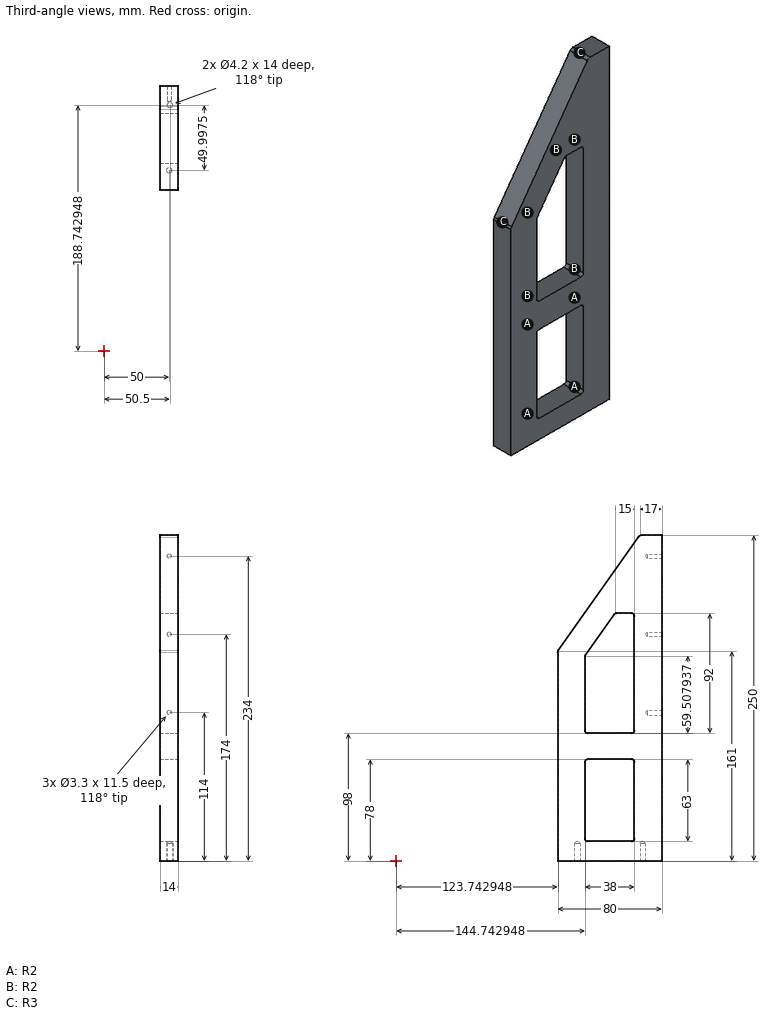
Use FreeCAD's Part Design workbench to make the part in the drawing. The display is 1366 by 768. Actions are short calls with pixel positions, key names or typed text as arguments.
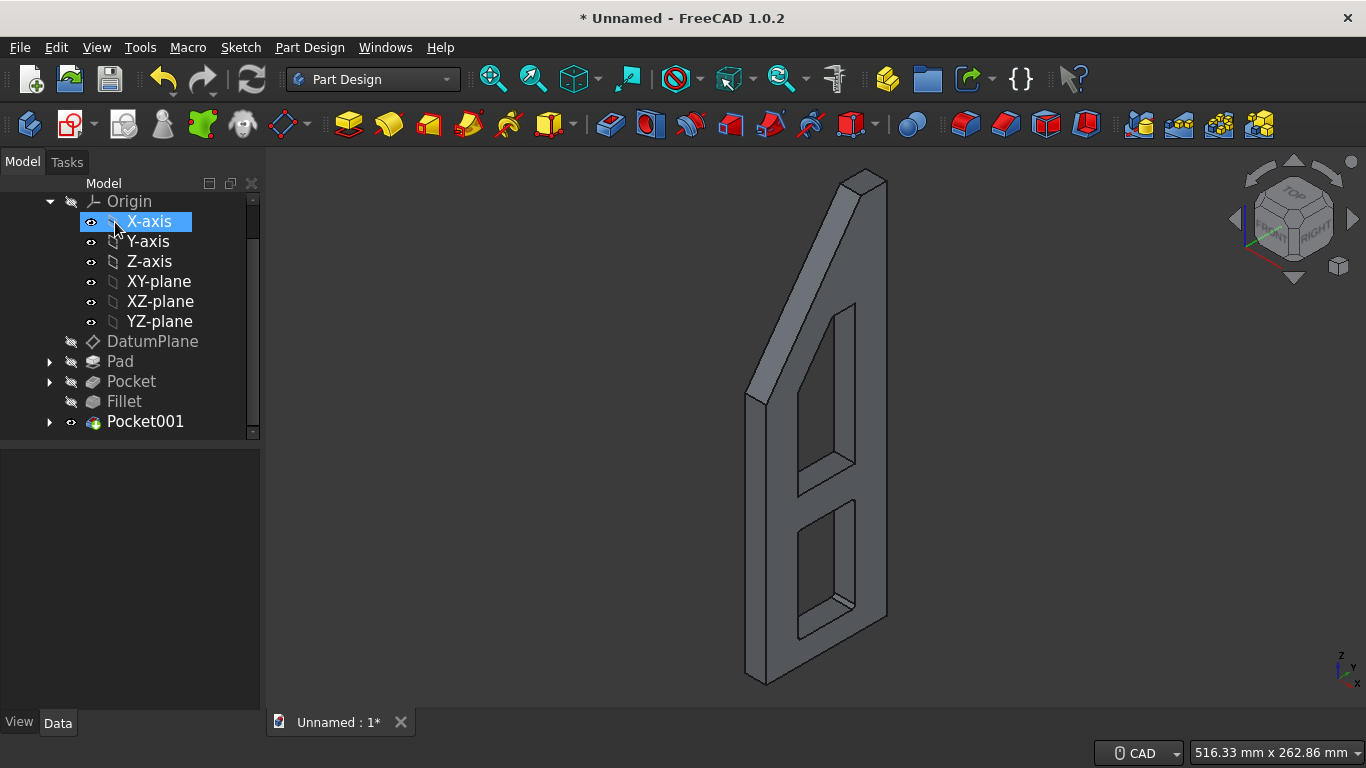
key(2)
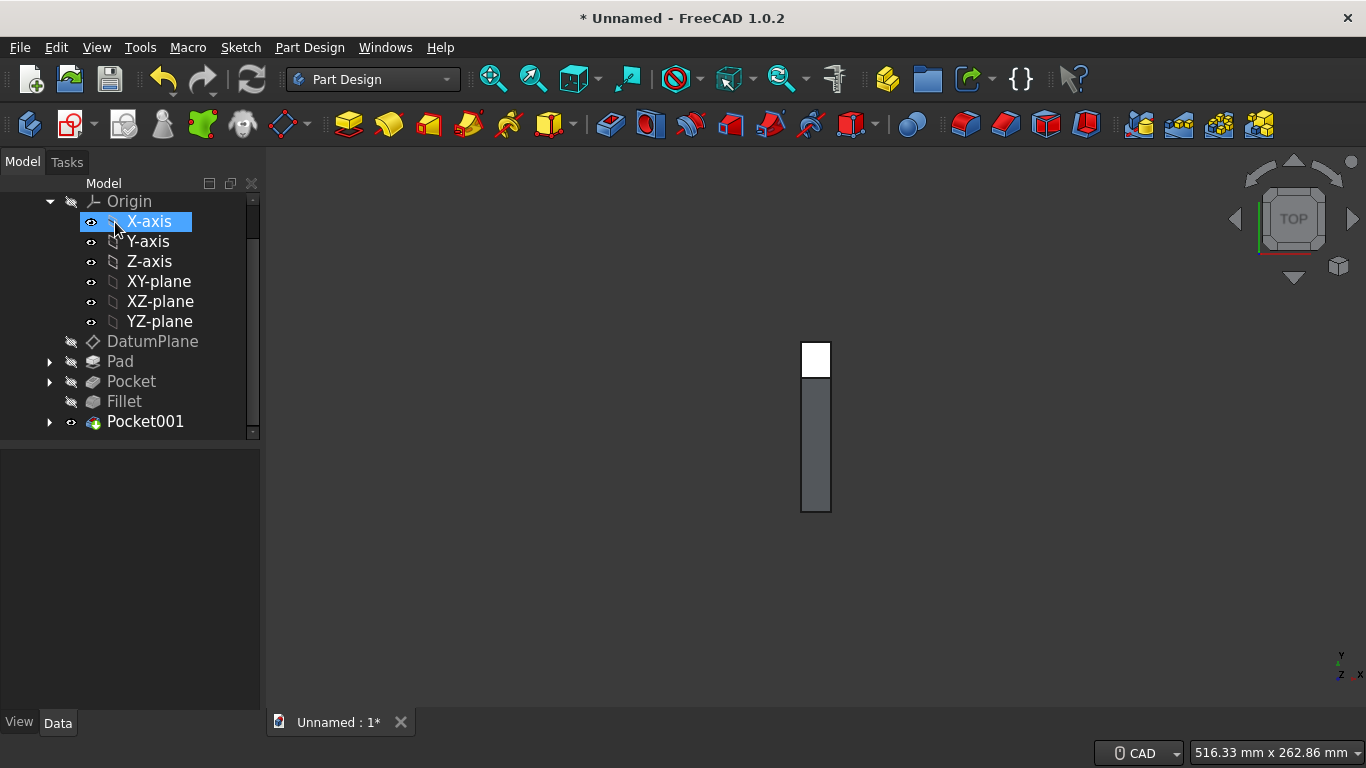
click(494, 80)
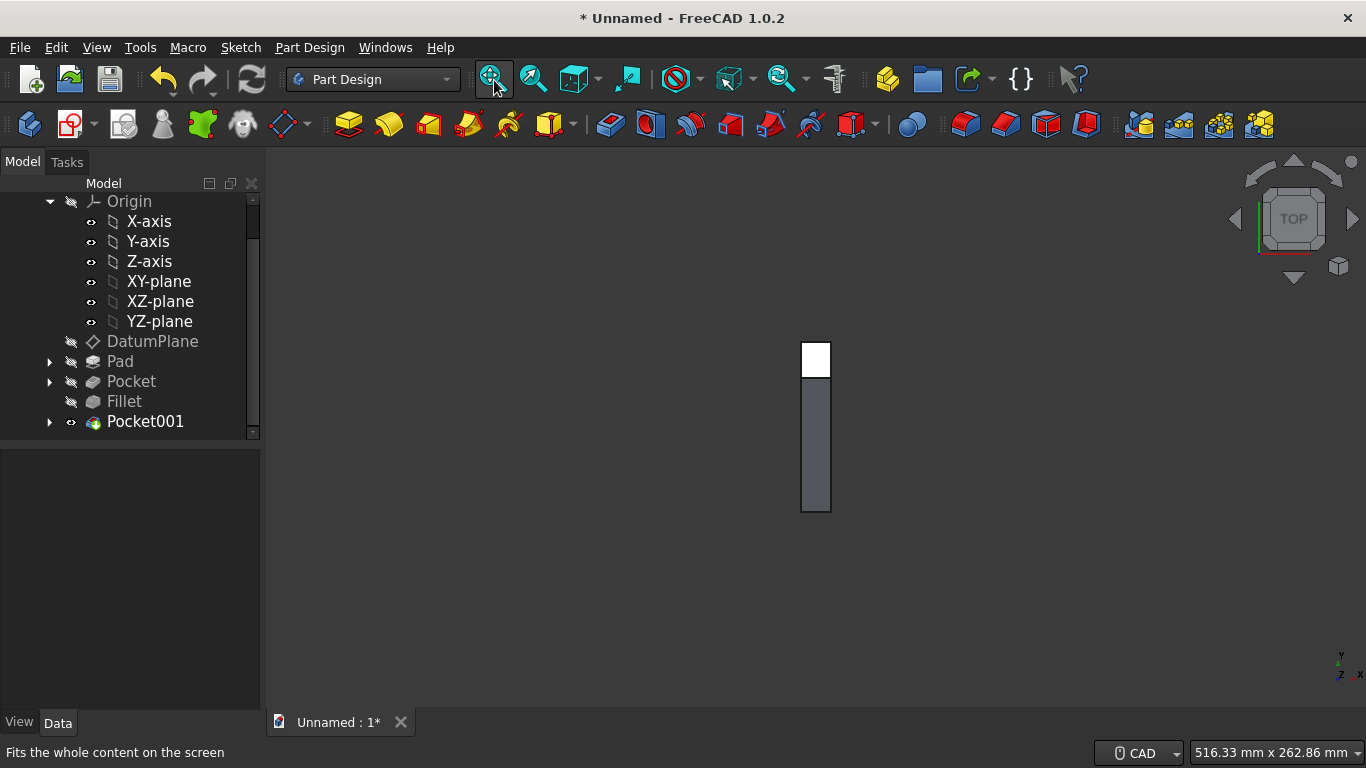
key(0)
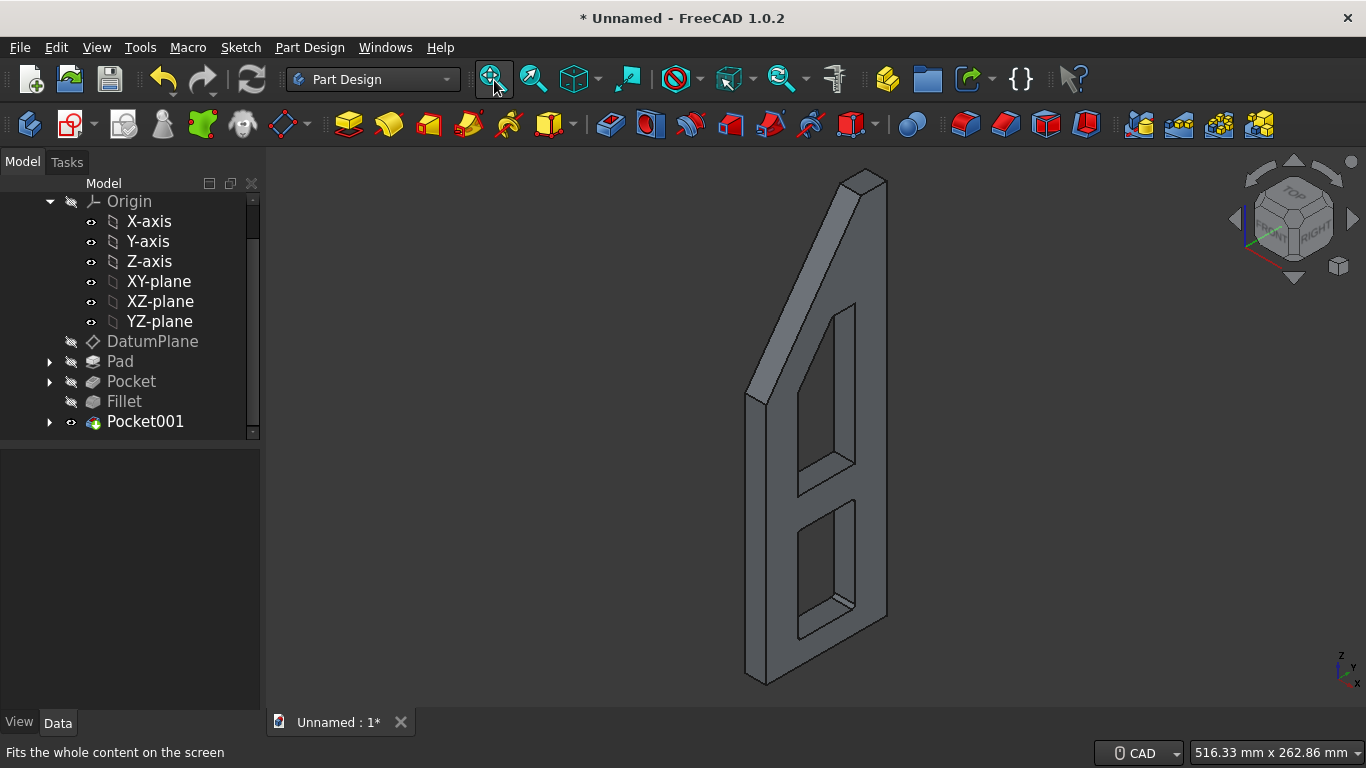
key(1)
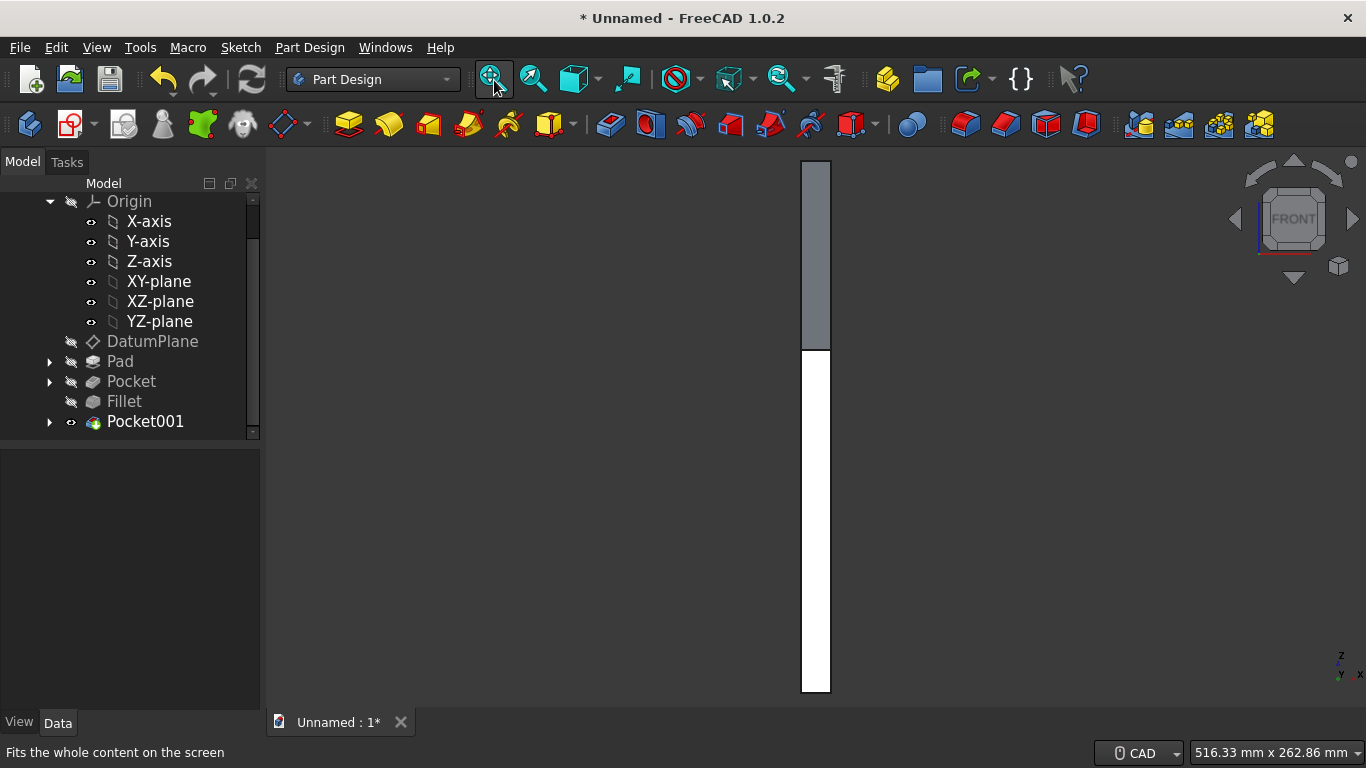
key(3)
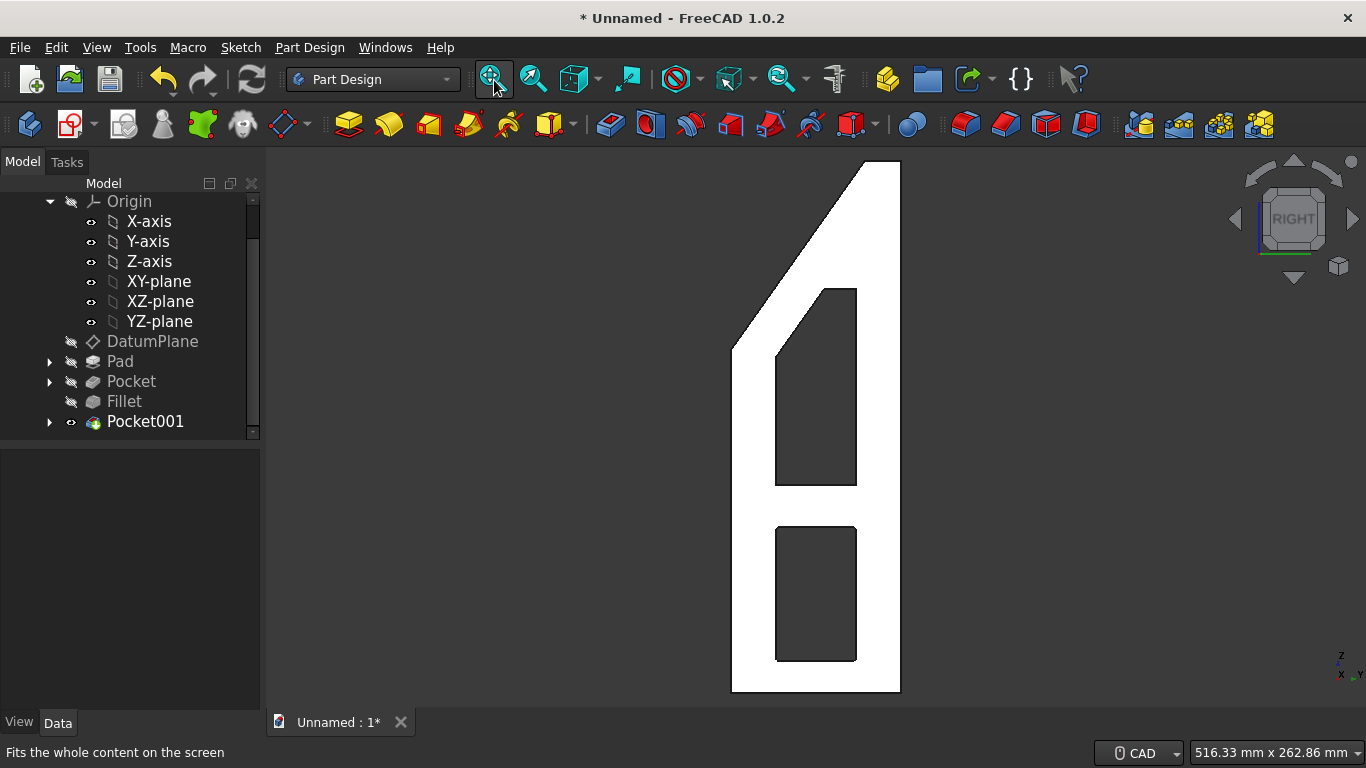
key(5)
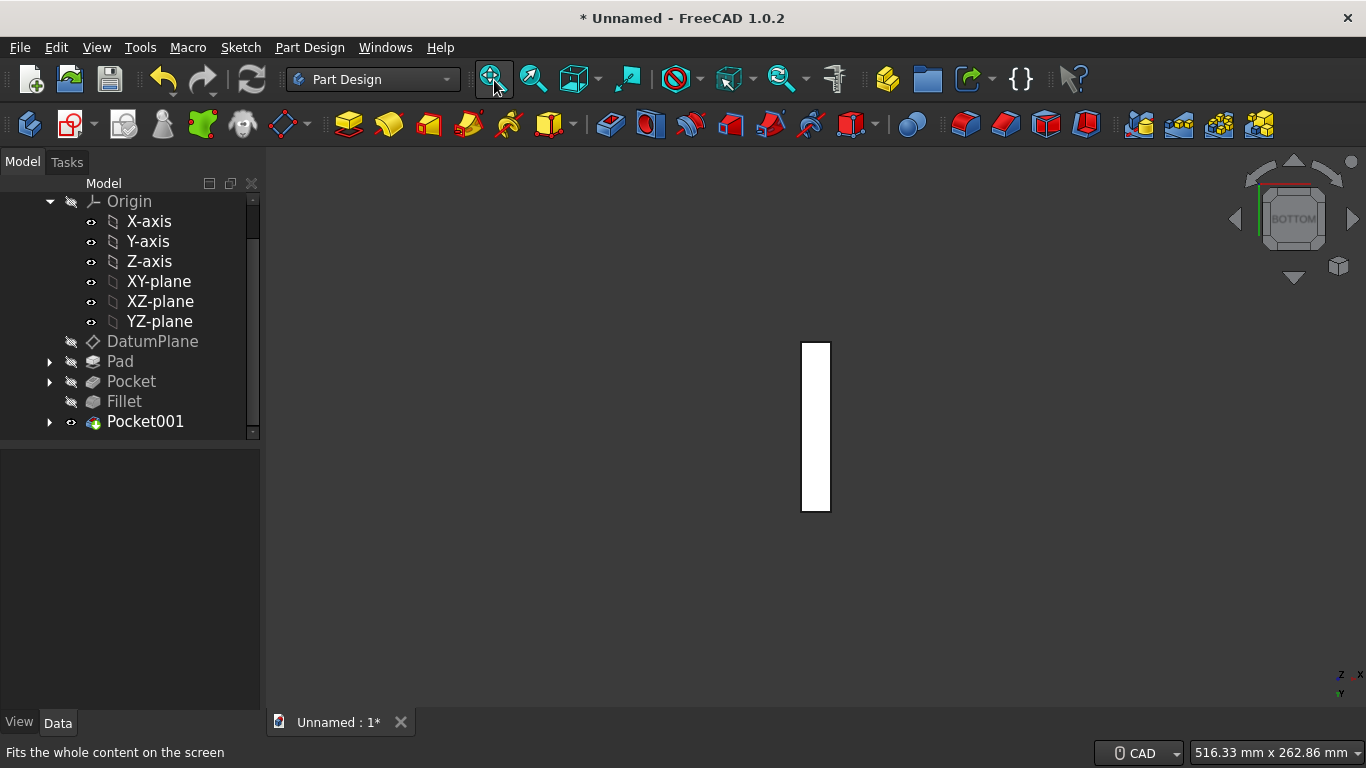
click(494, 80)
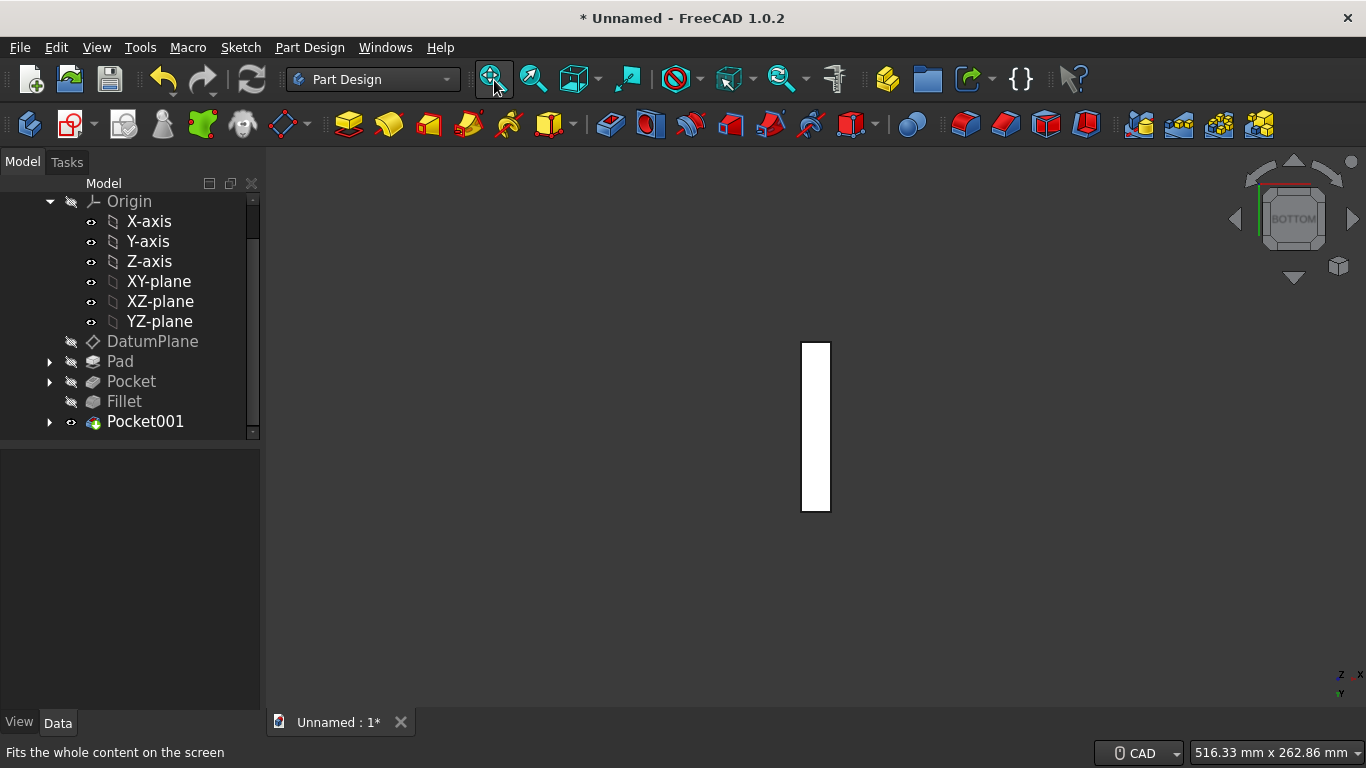
key(4)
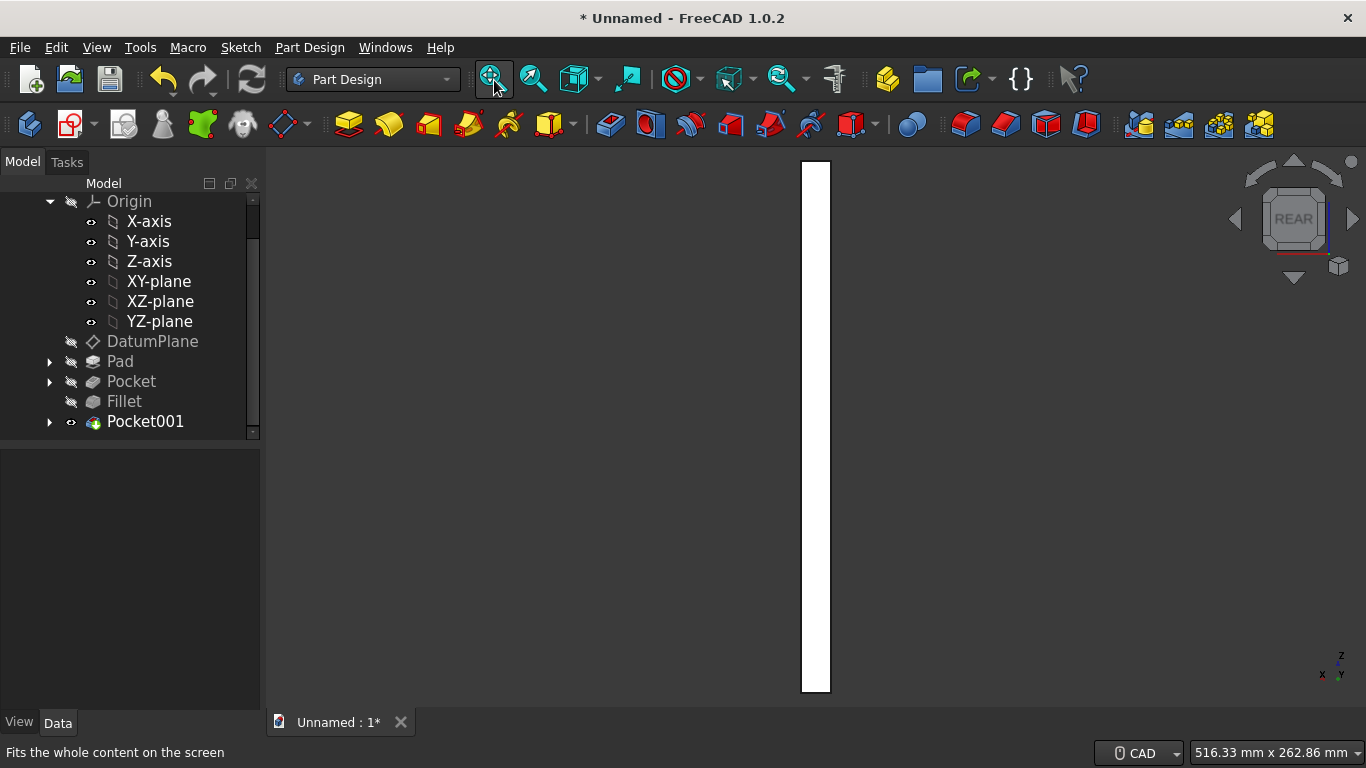
key(6)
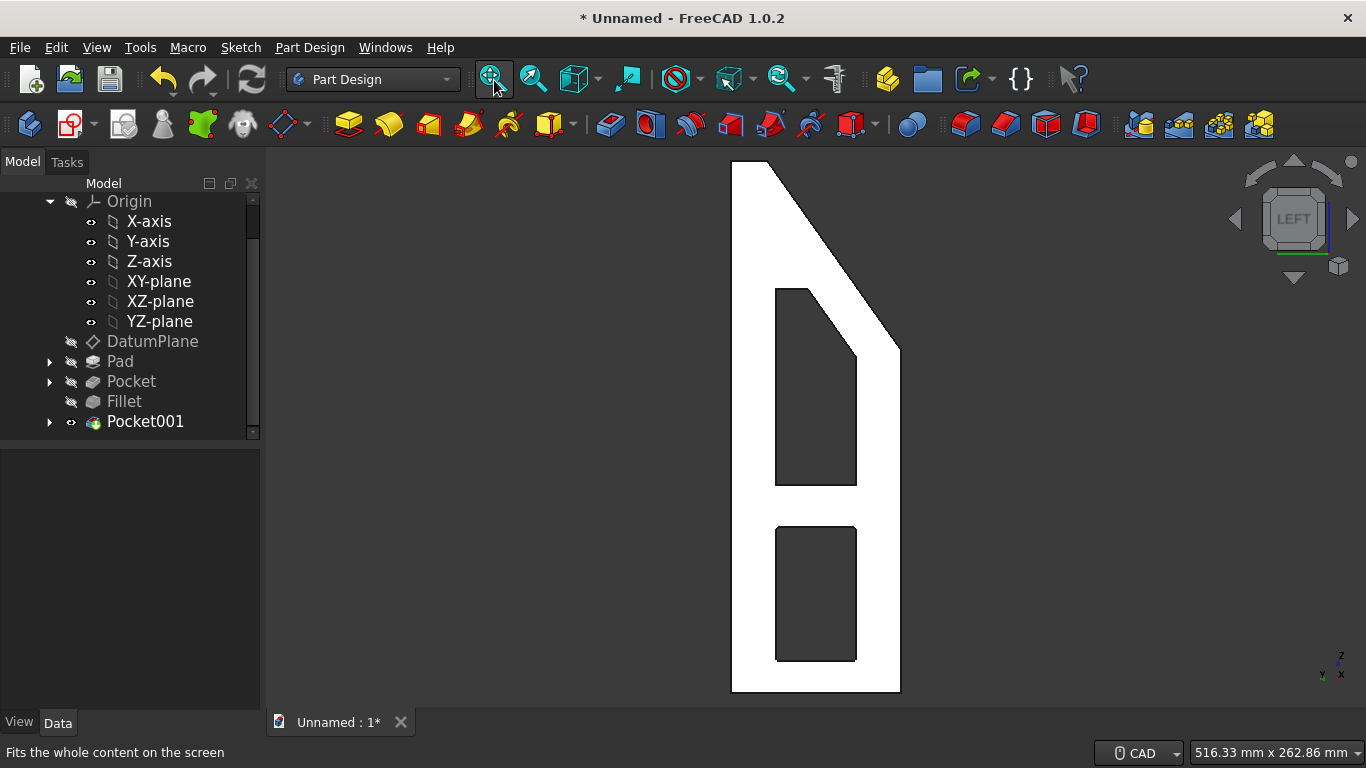
key(v)
key(3)